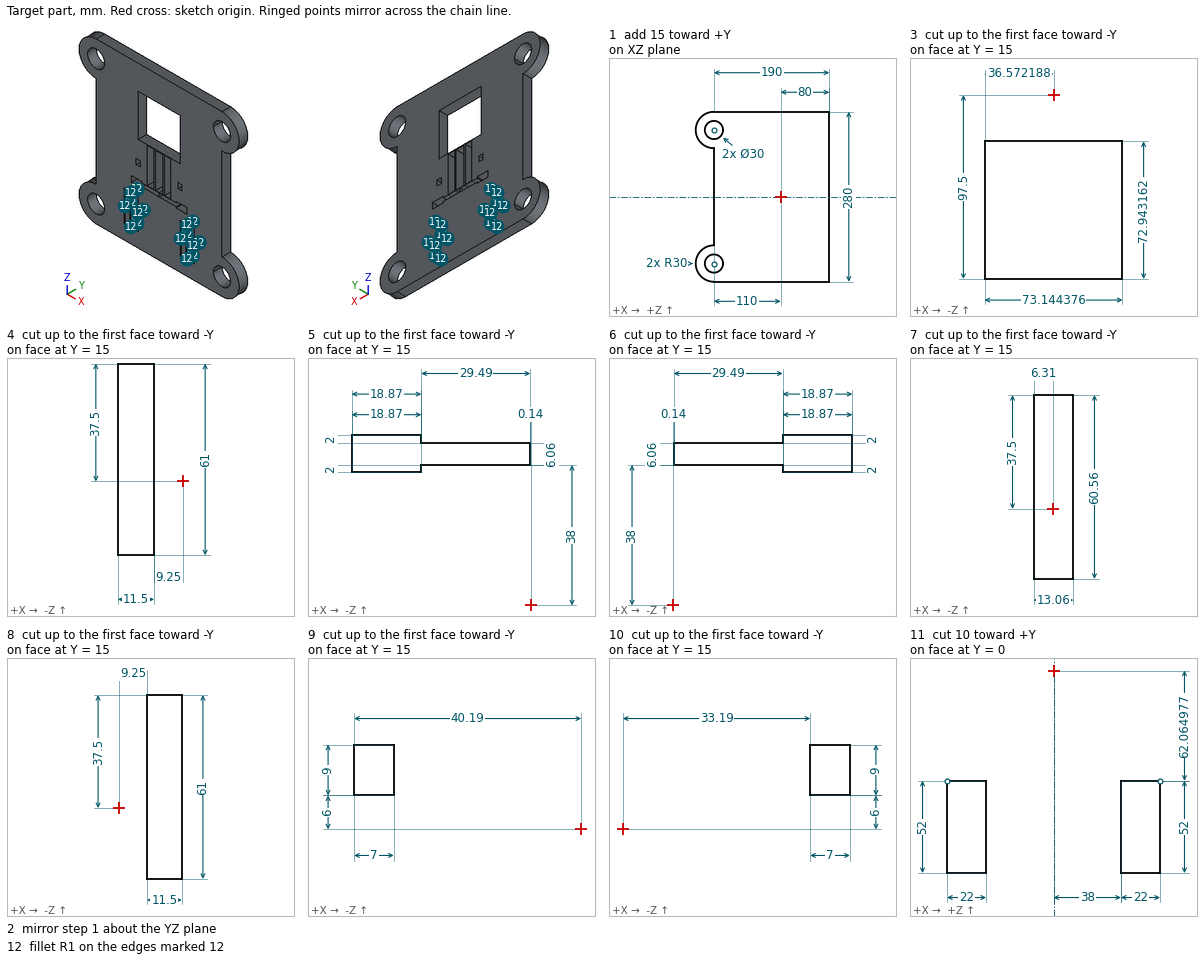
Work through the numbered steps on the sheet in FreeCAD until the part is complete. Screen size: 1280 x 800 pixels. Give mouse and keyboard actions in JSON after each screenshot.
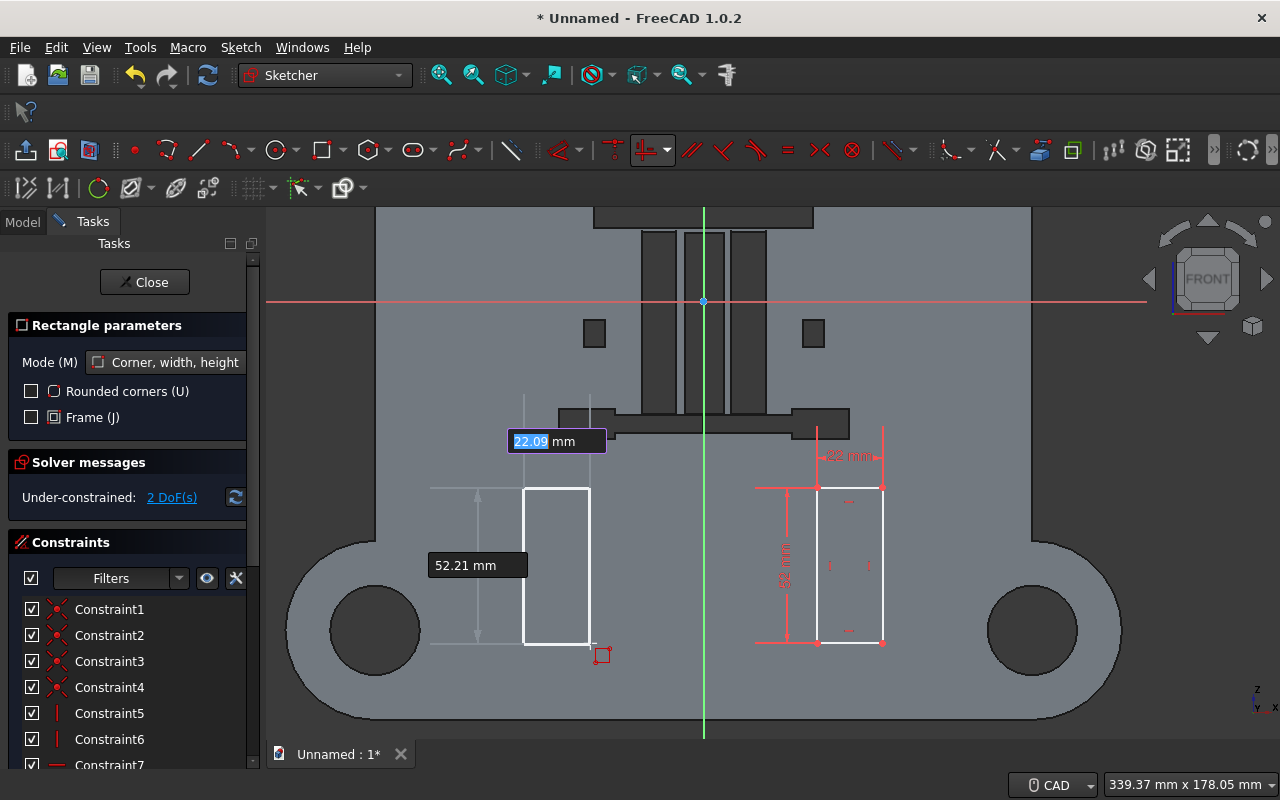
{"action": "type", "text": "22"}
{"action": "key", "text": "Tab"}
{"action": "type", "text": "52"}
{"action": "key", "text": "Return"}
{"action": "key", "text": "Escape"}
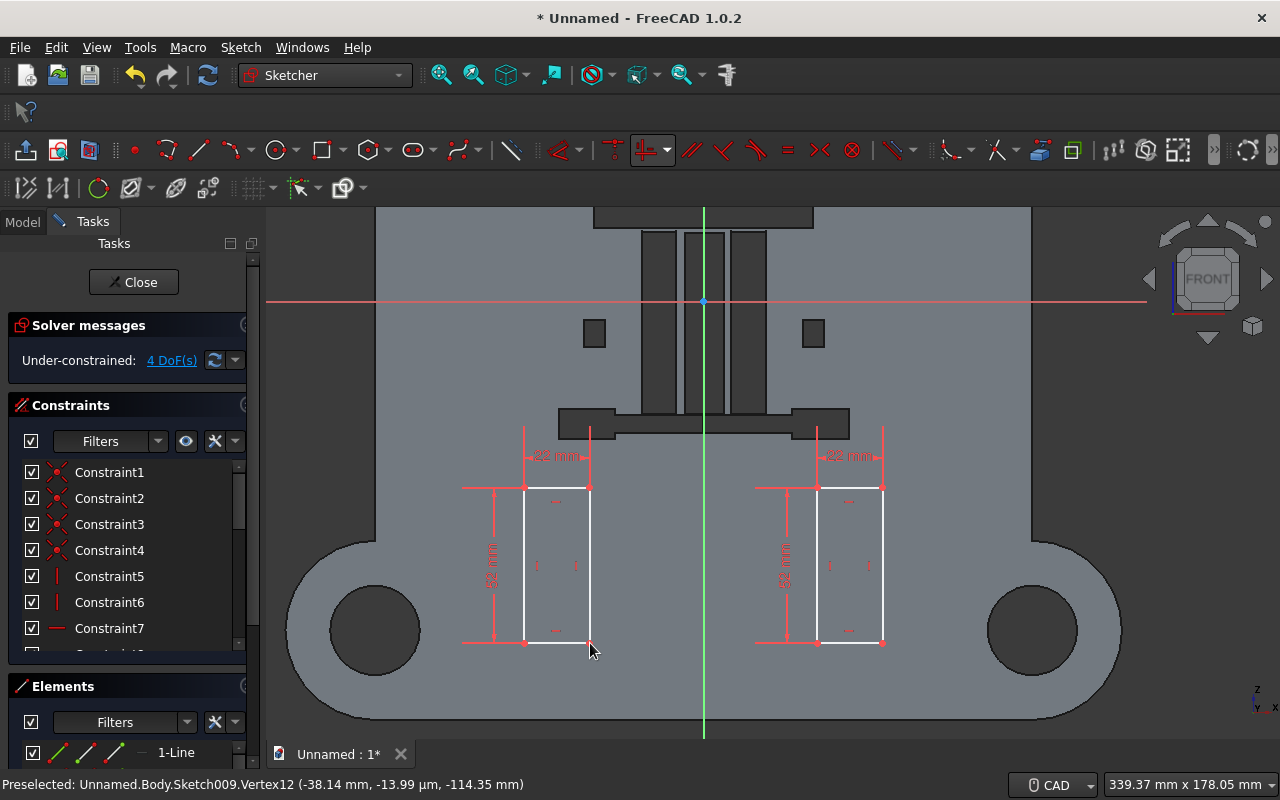
{"action": "left_click", "coordinate": [883, 488]}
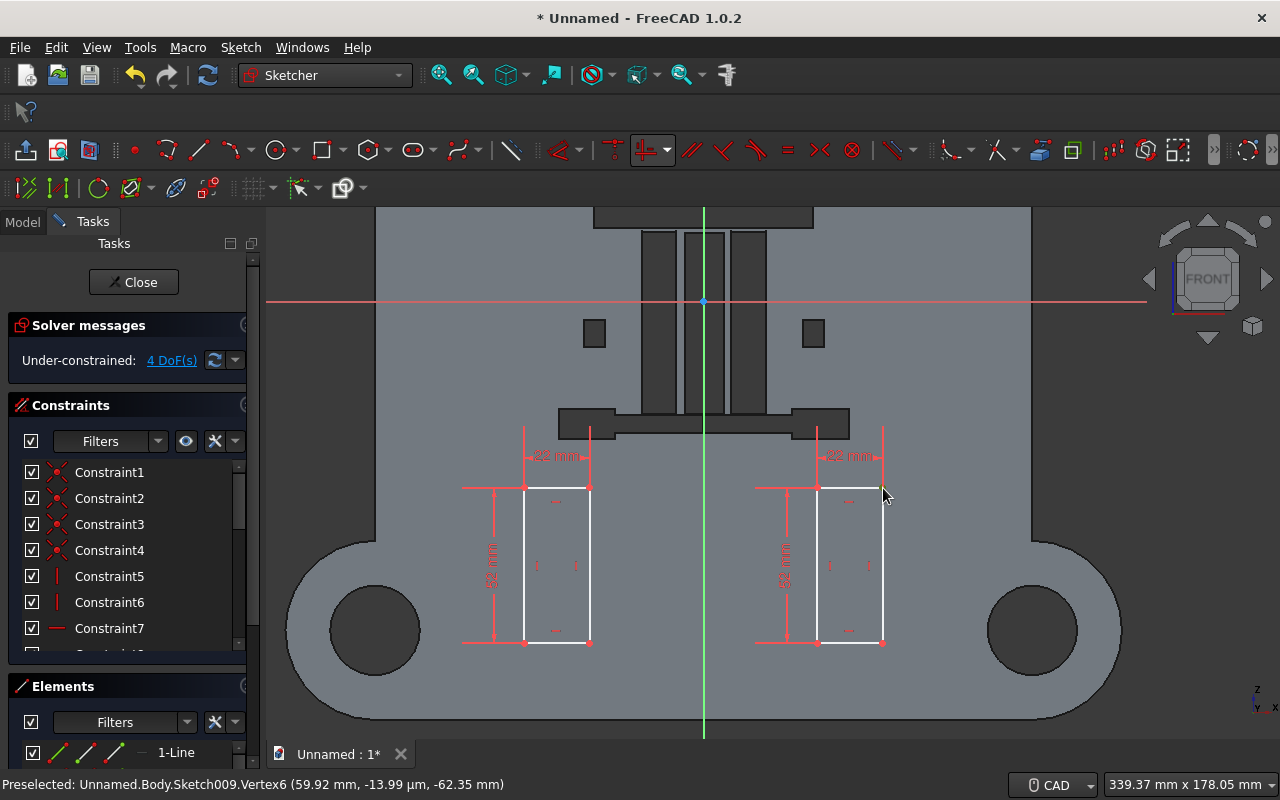
{"action": "left_click", "coordinate": [524, 488]}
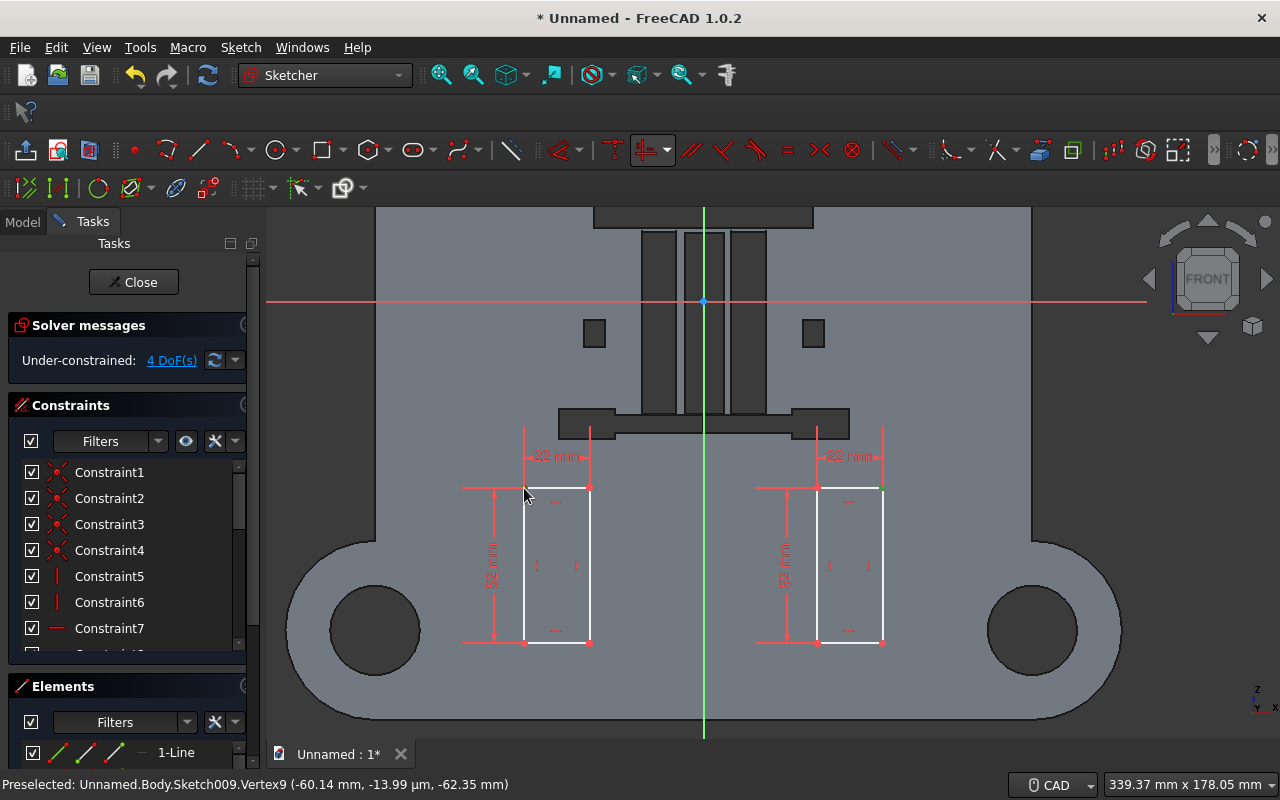
{"action": "left_click", "coordinate": [704, 677]}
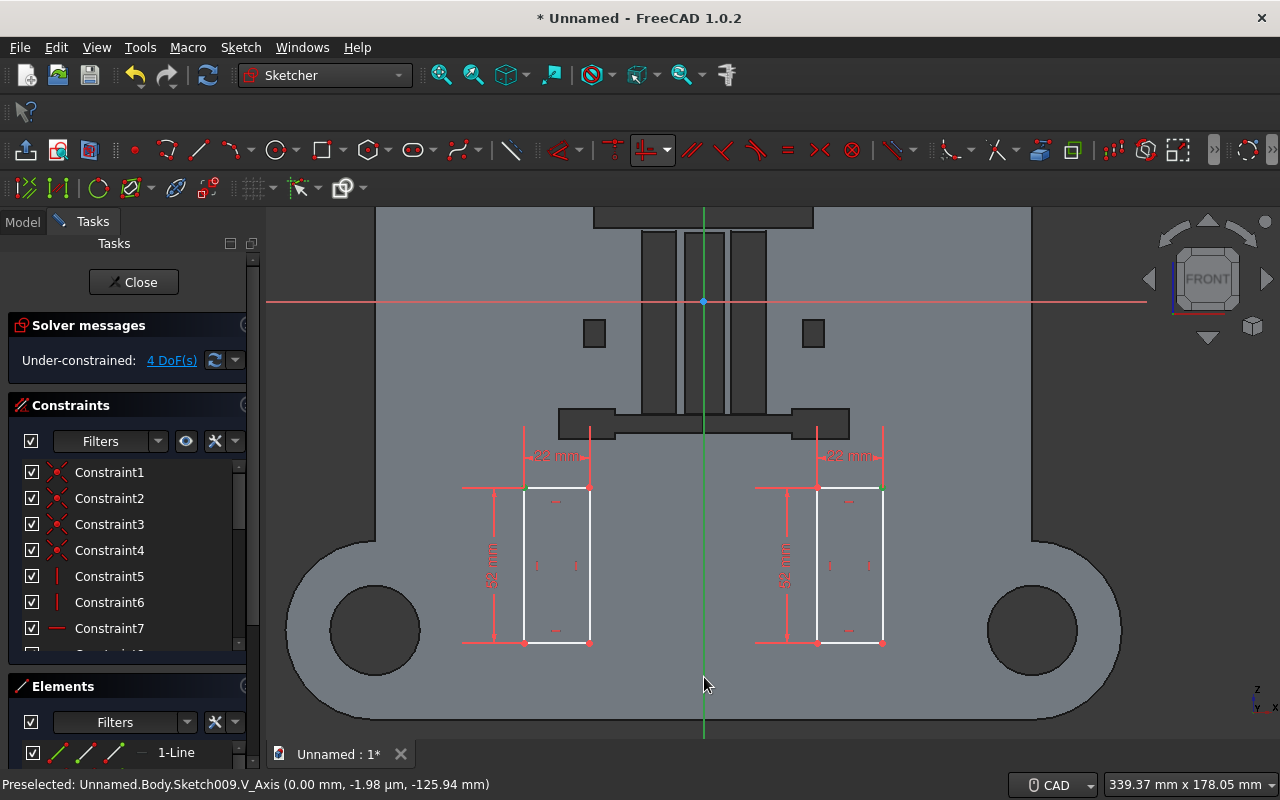
{"action": "key", "text": "s"}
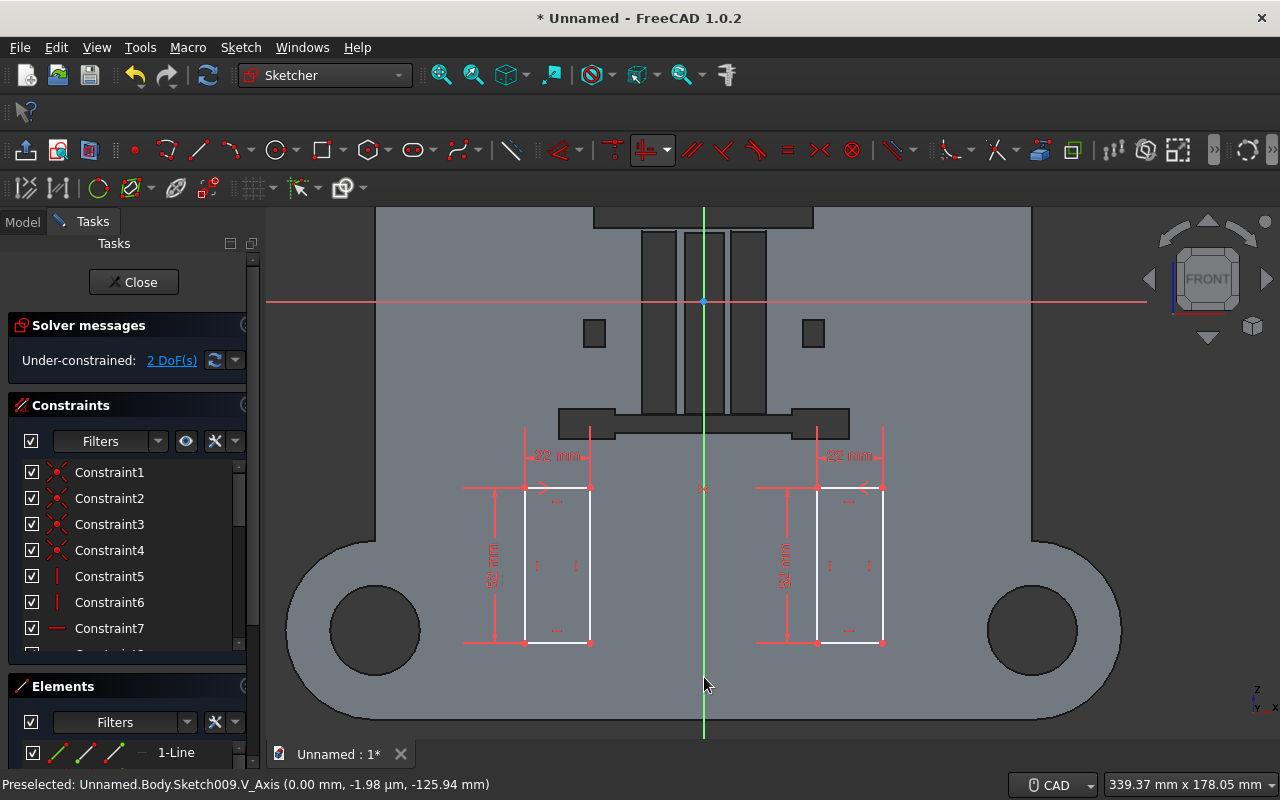
{"action": "left_click", "coordinate": [558, 150]}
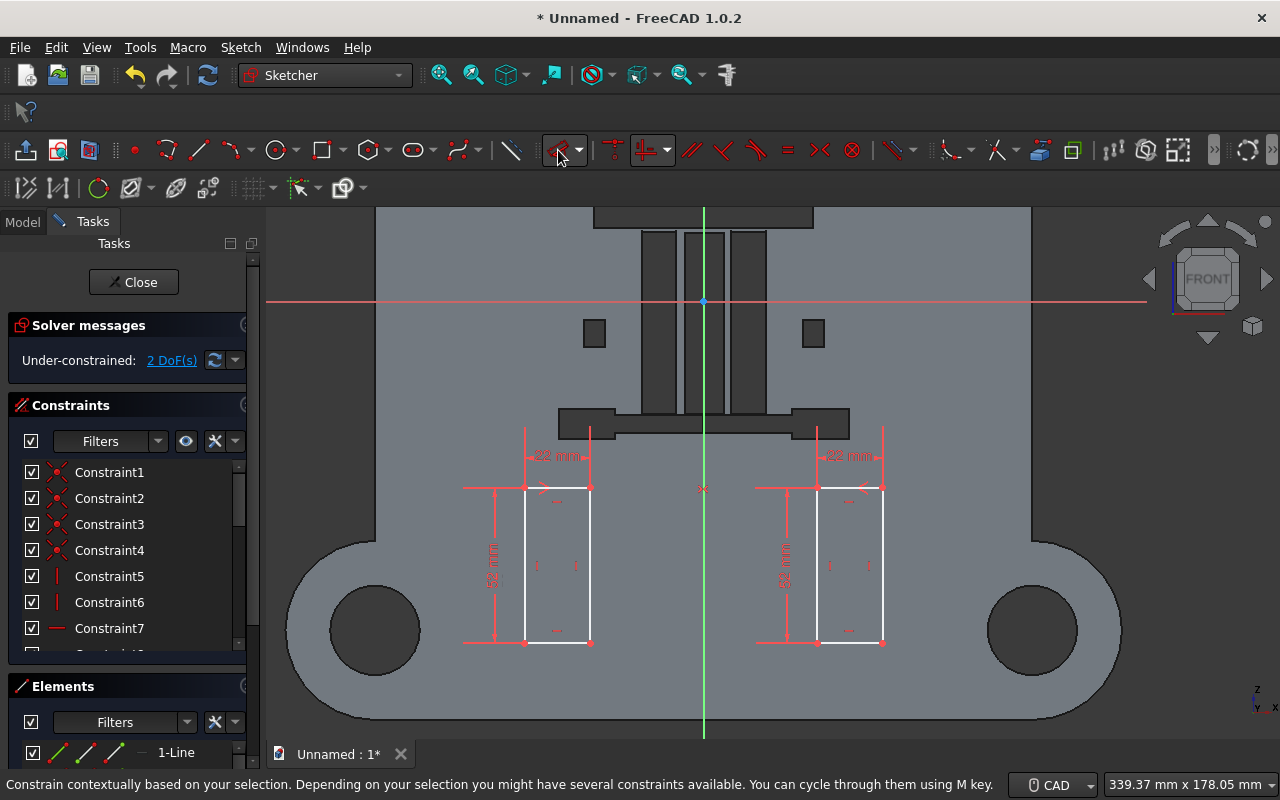
{"action": "left_click", "coordinate": [817, 488]}
{"action": "left_click", "coordinate": [760, 268]}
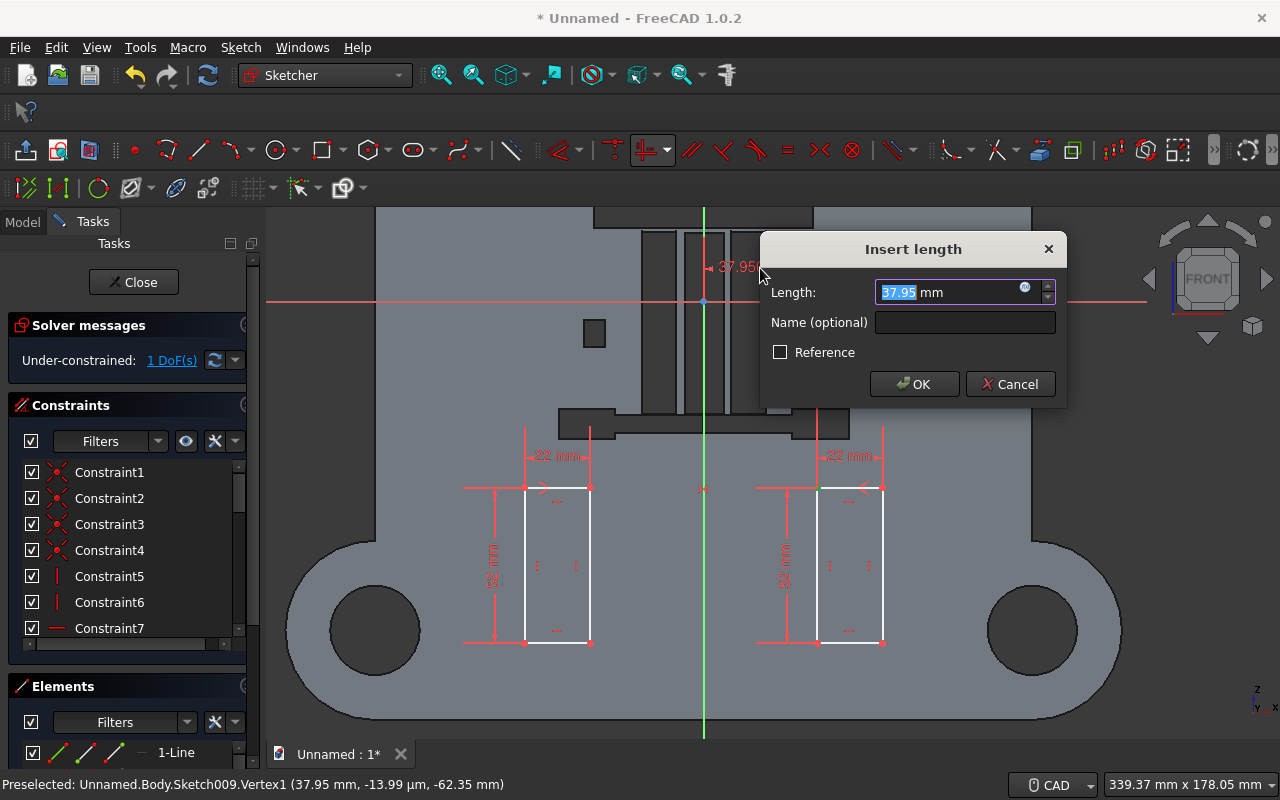
{"action": "type", "text": "38"}
{"action": "key", "text": "Return"}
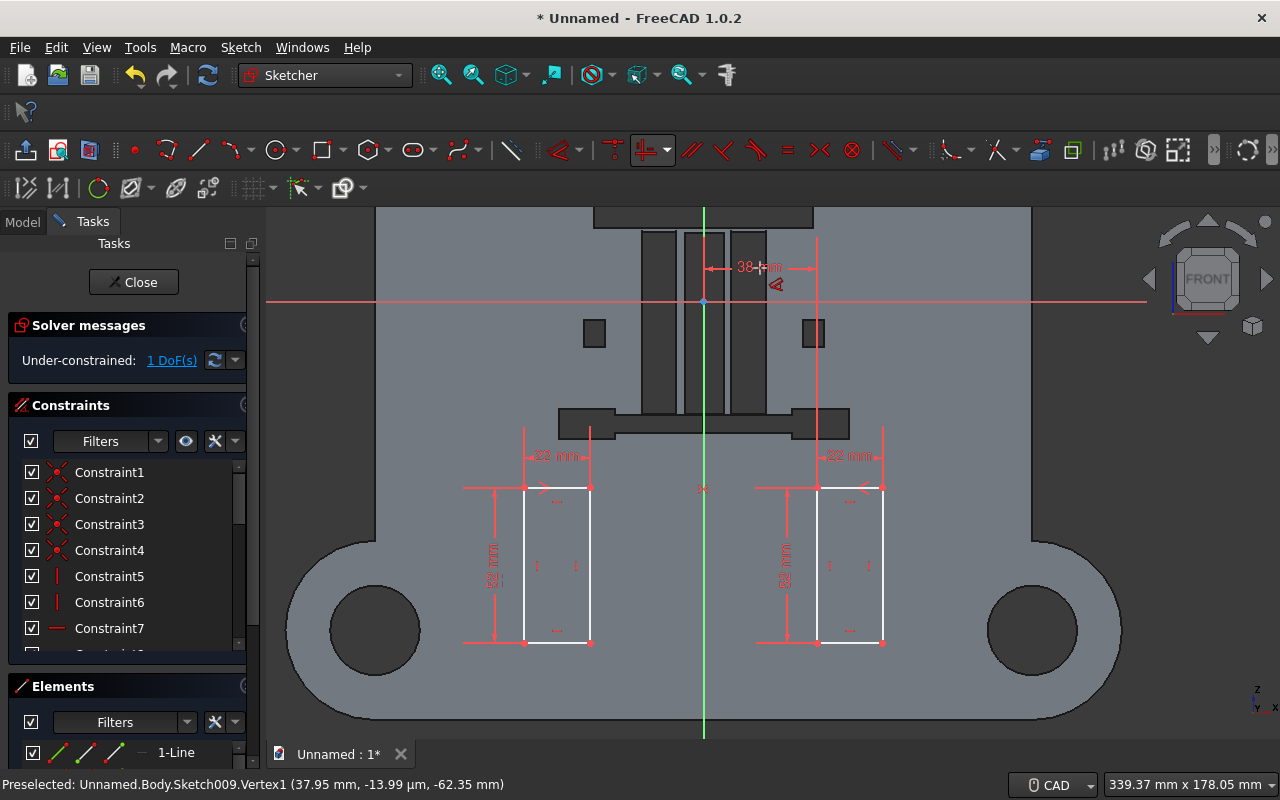
{"action": "left_click", "coordinate": [817, 488]}
{"action": "left_click", "coordinate": [851, 395]}